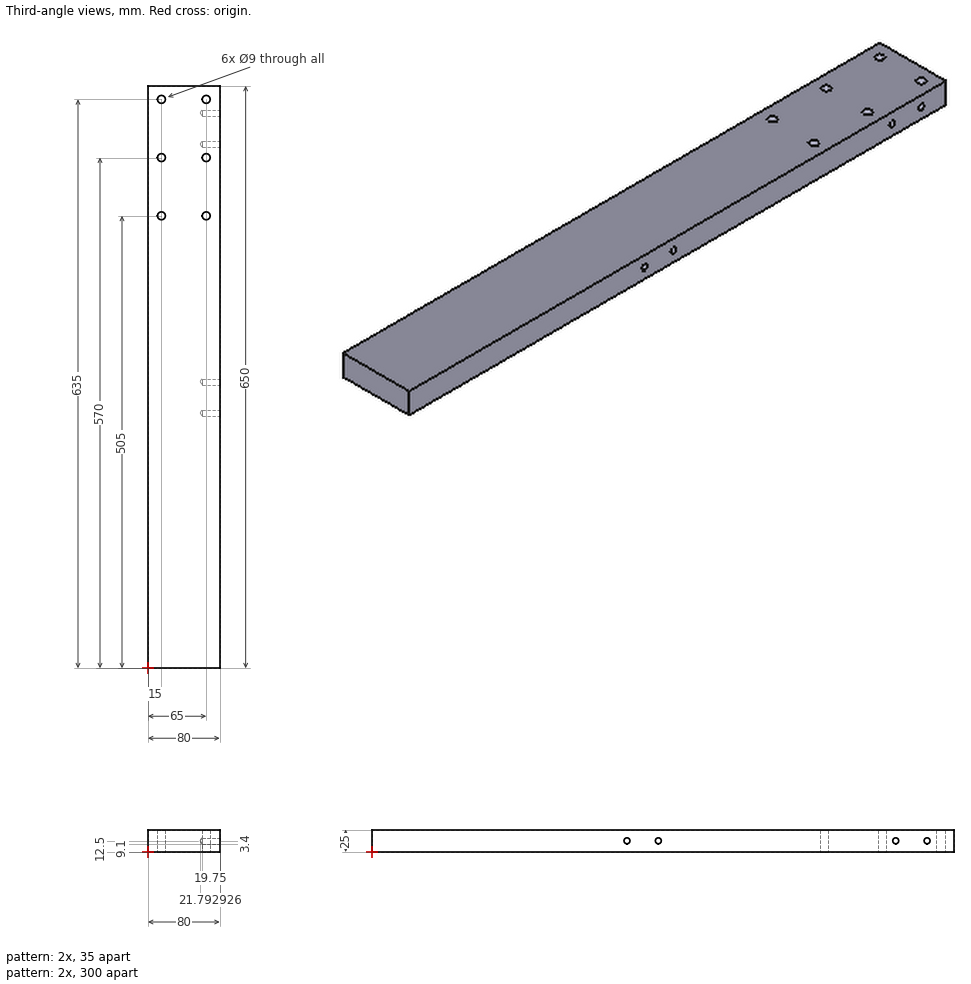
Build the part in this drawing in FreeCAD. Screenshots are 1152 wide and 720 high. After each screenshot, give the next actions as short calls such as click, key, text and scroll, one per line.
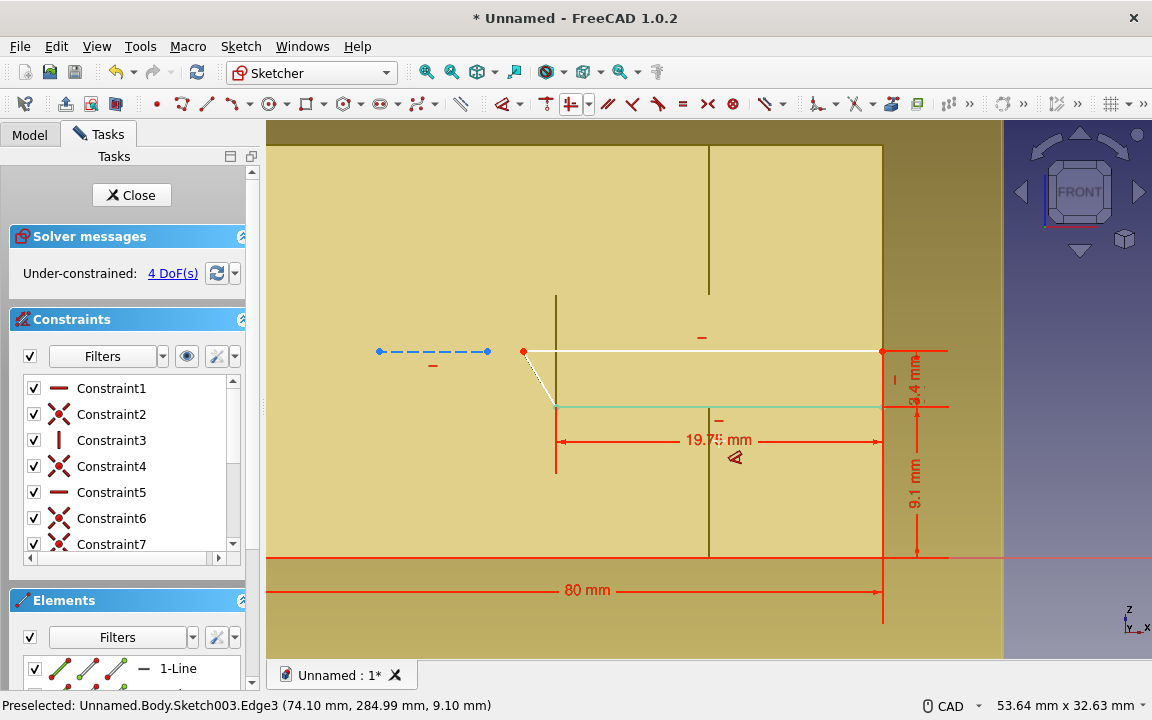
click(487, 352)
click(521, 455)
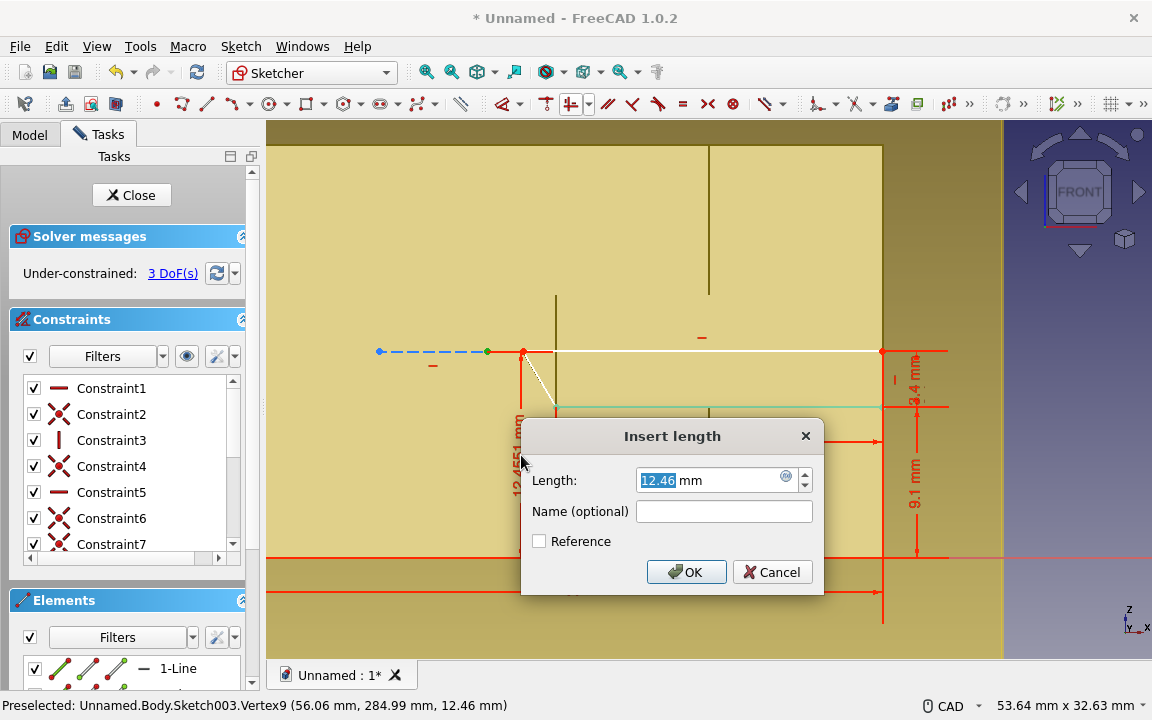
text(12.5)
key(Return)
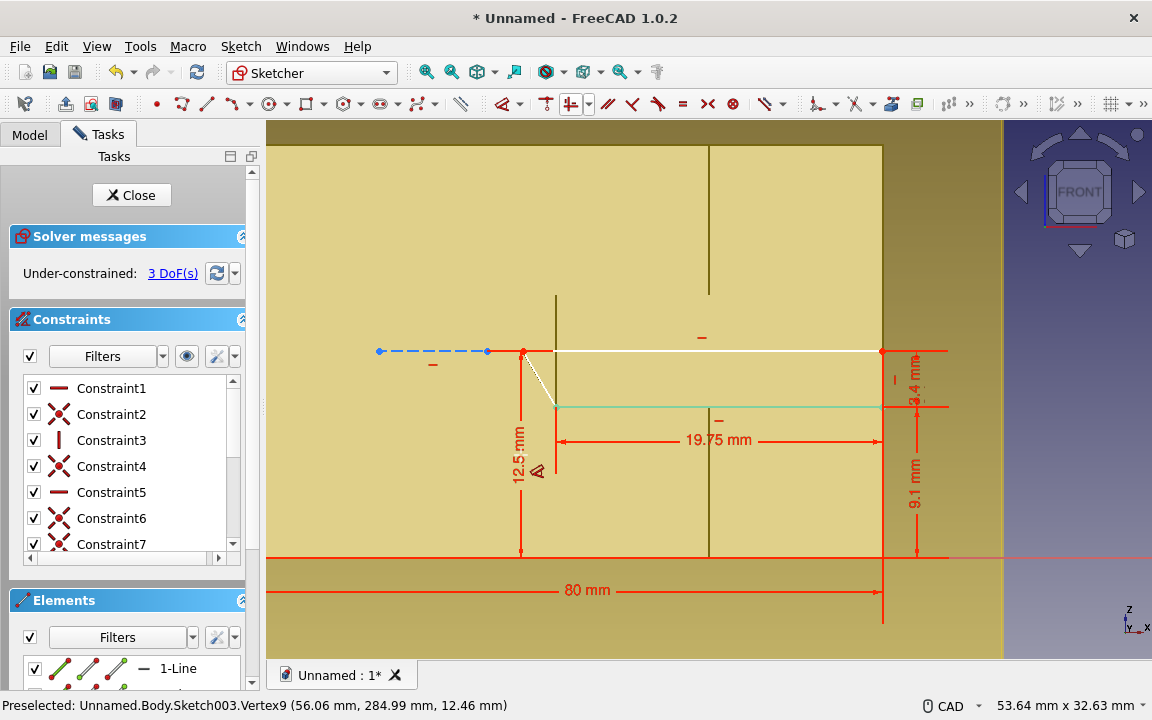
click(631, 351)
click(703, 317)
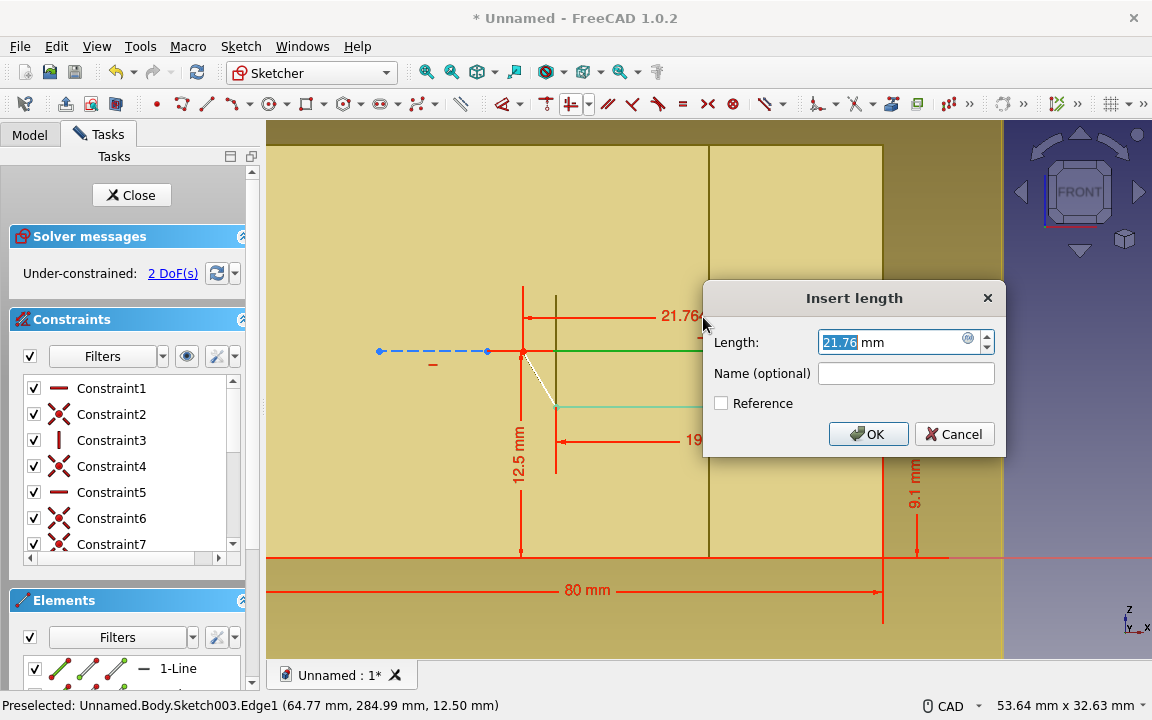
text(21.792926)
key(Return)
key(Escape)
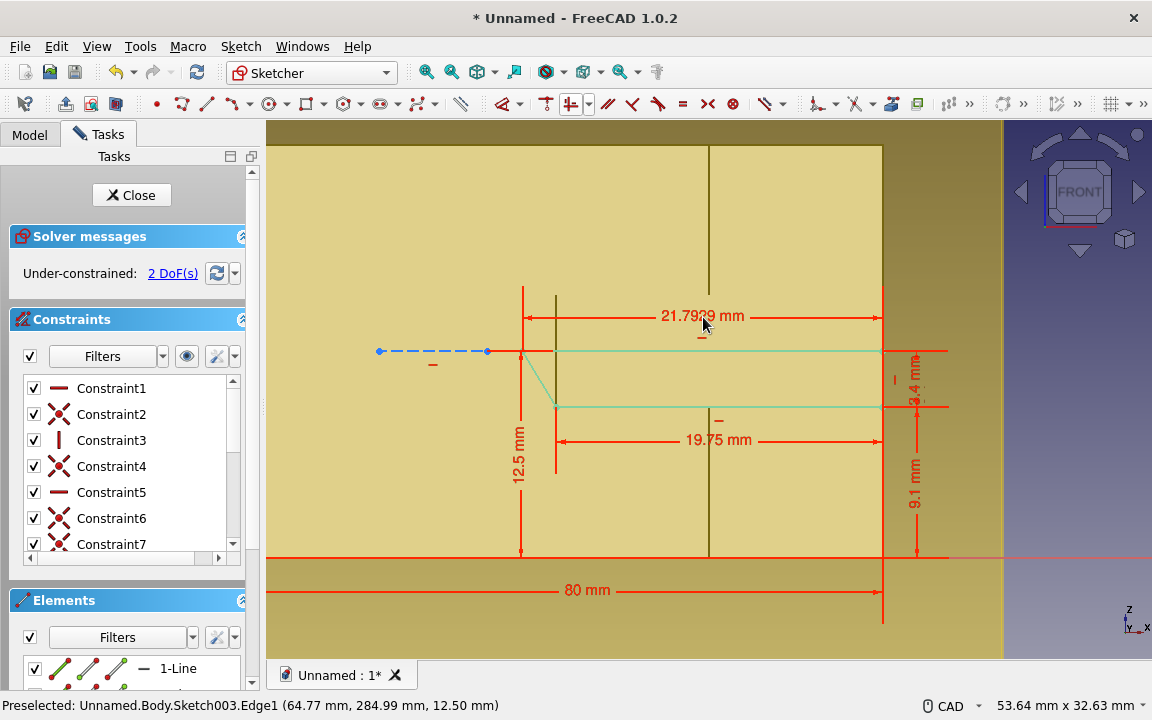
click(132, 195)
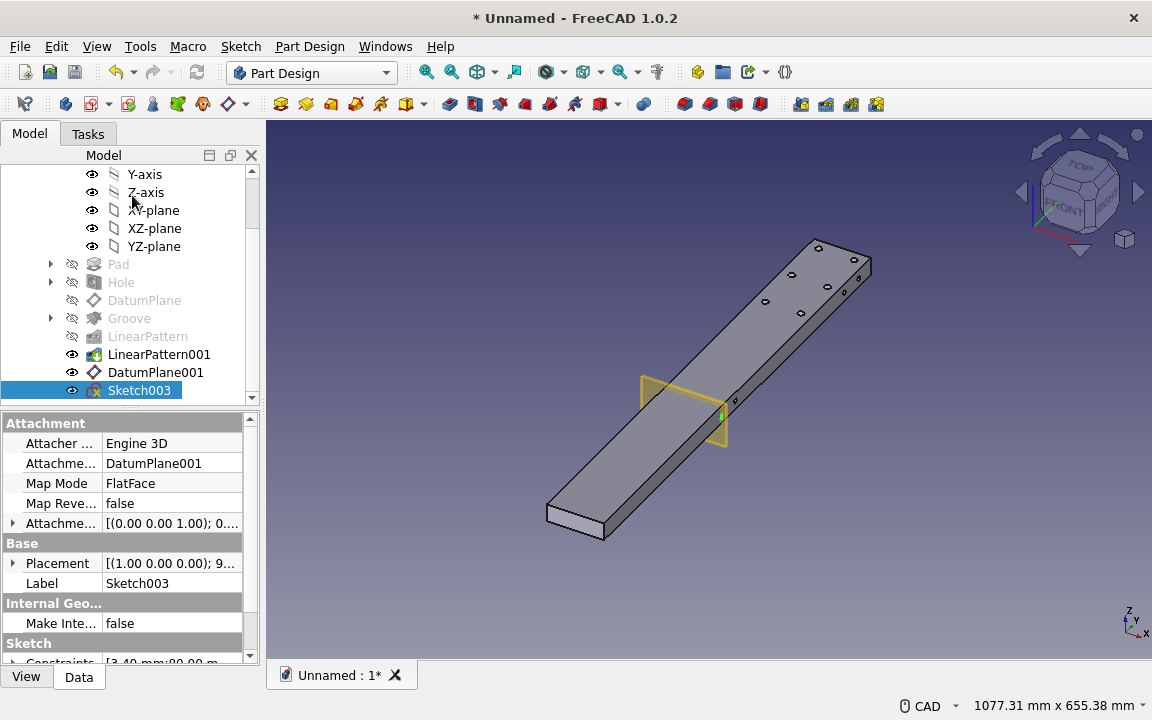
click(500, 104)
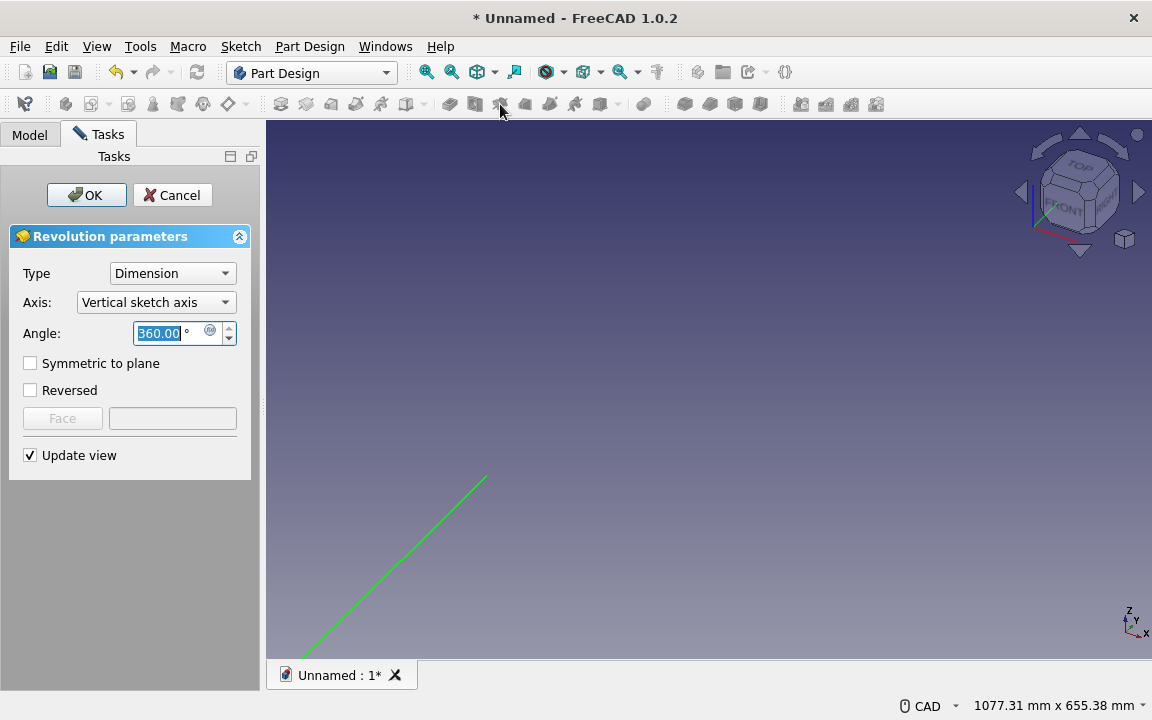
click(157, 302)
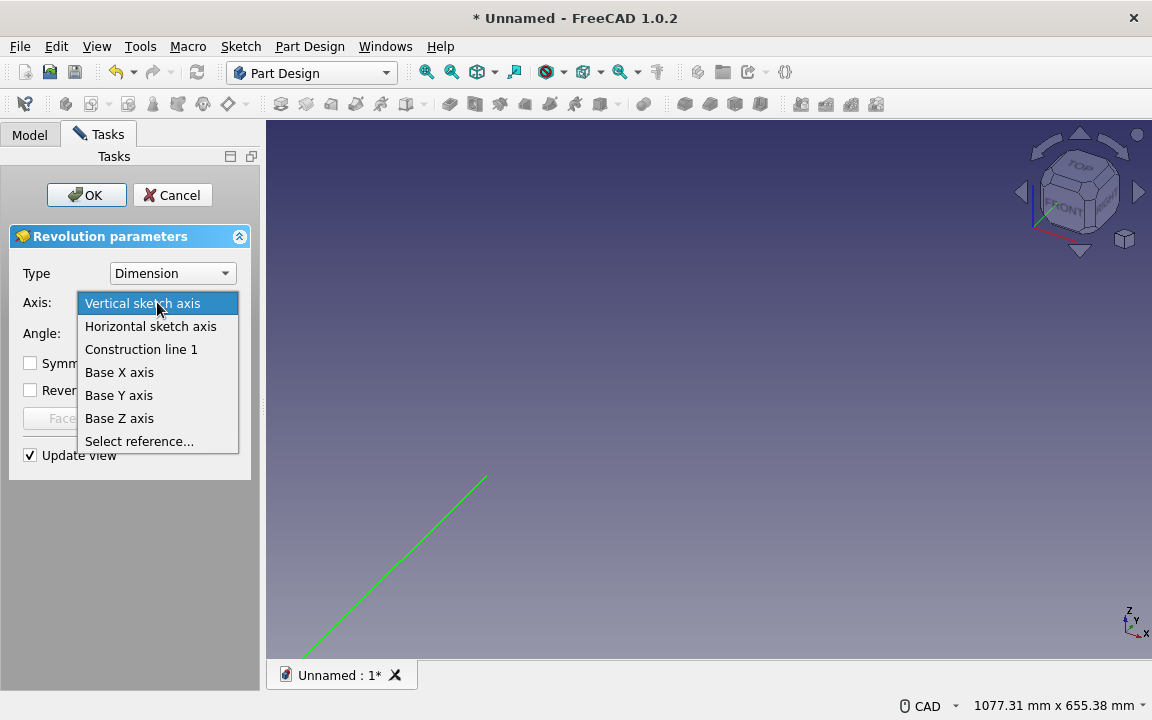
click(156, 350)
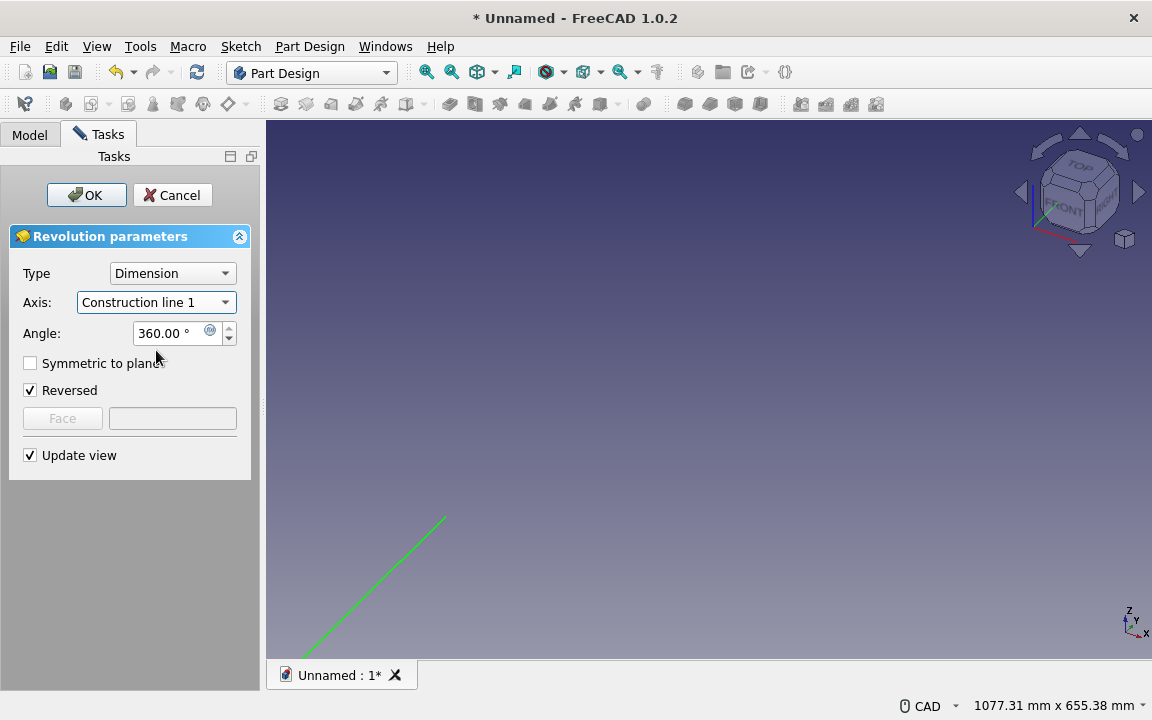
click(87, 195)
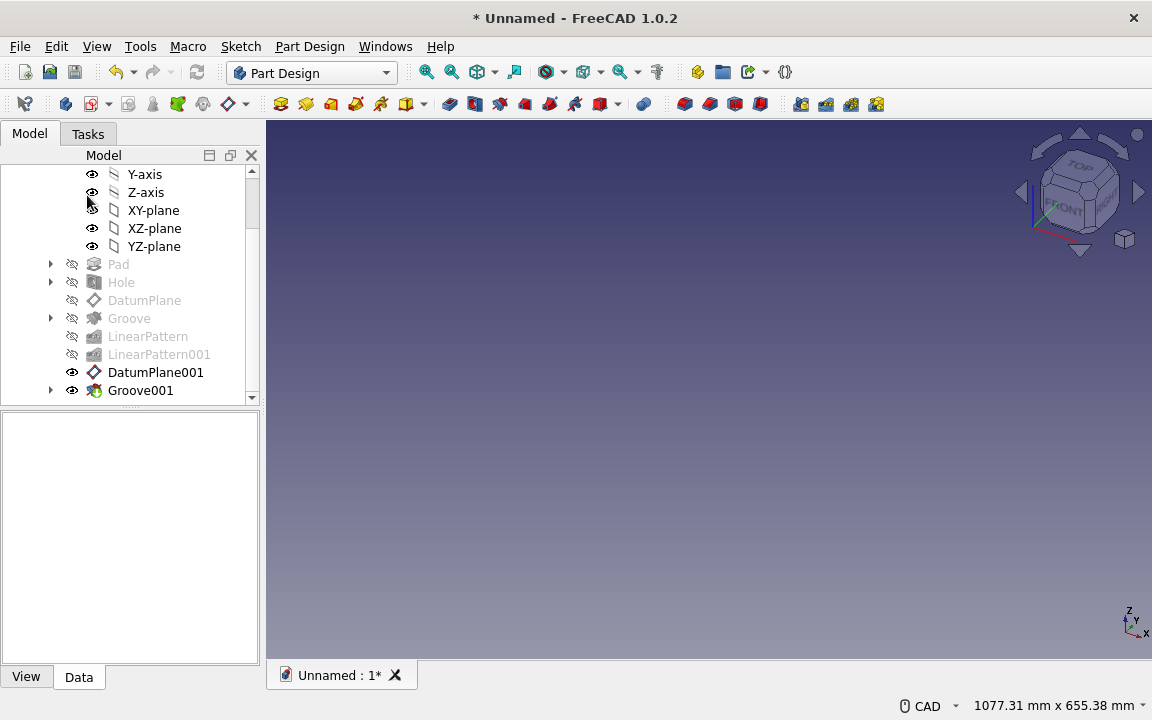
click(117, 372)
key(space)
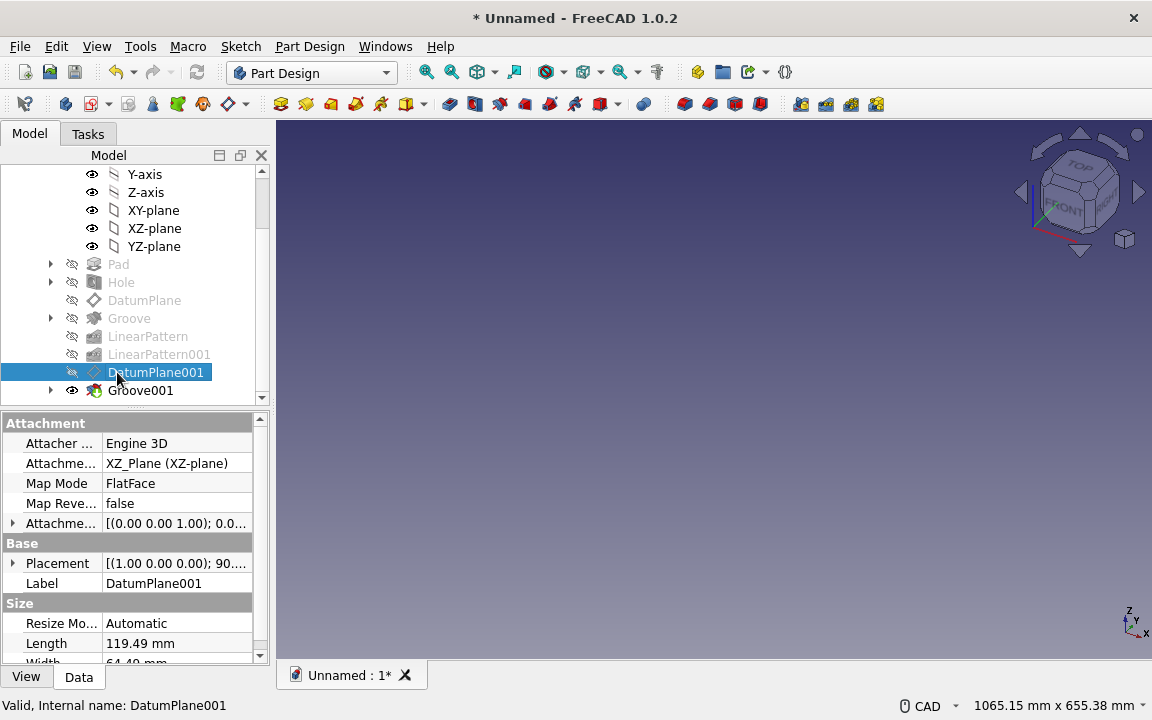
key(0)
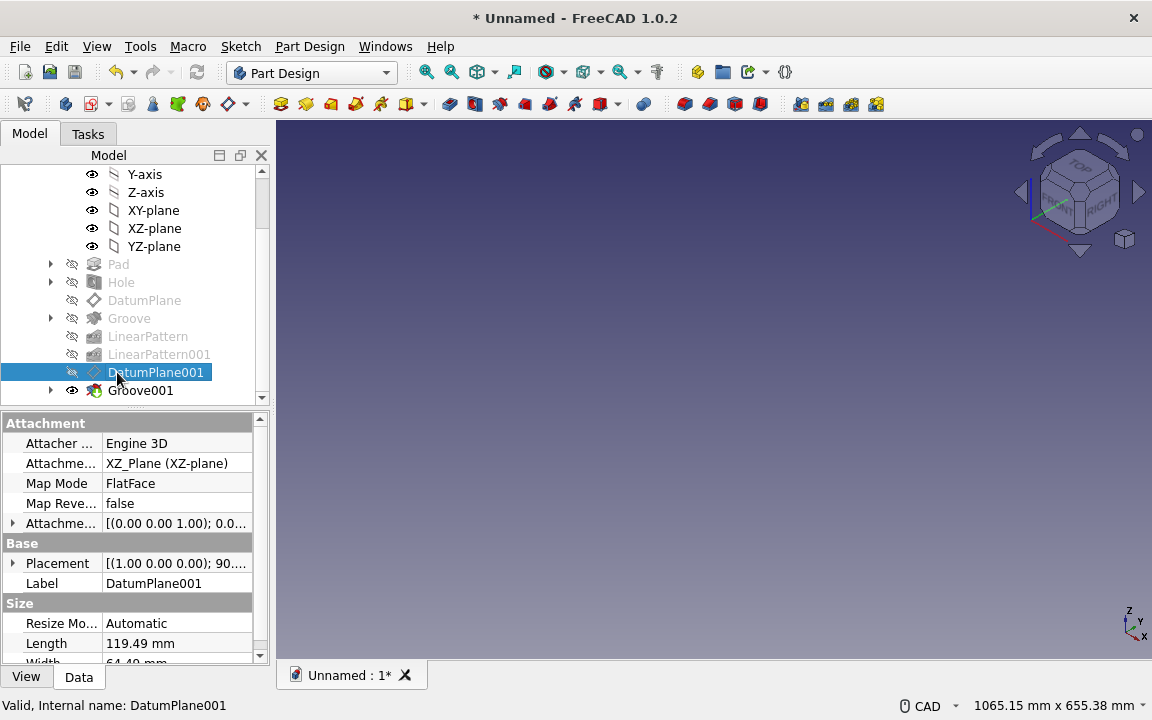
click(427, 72)